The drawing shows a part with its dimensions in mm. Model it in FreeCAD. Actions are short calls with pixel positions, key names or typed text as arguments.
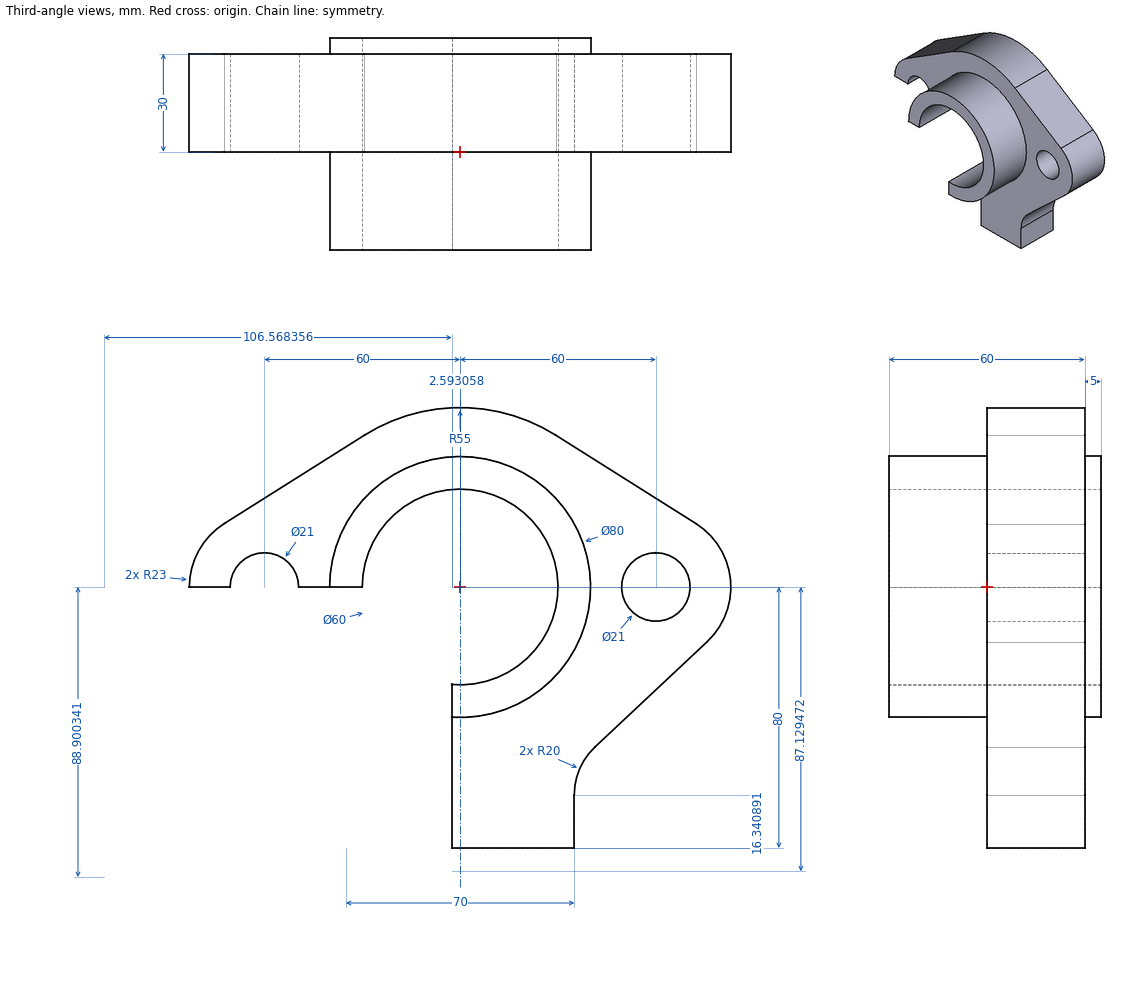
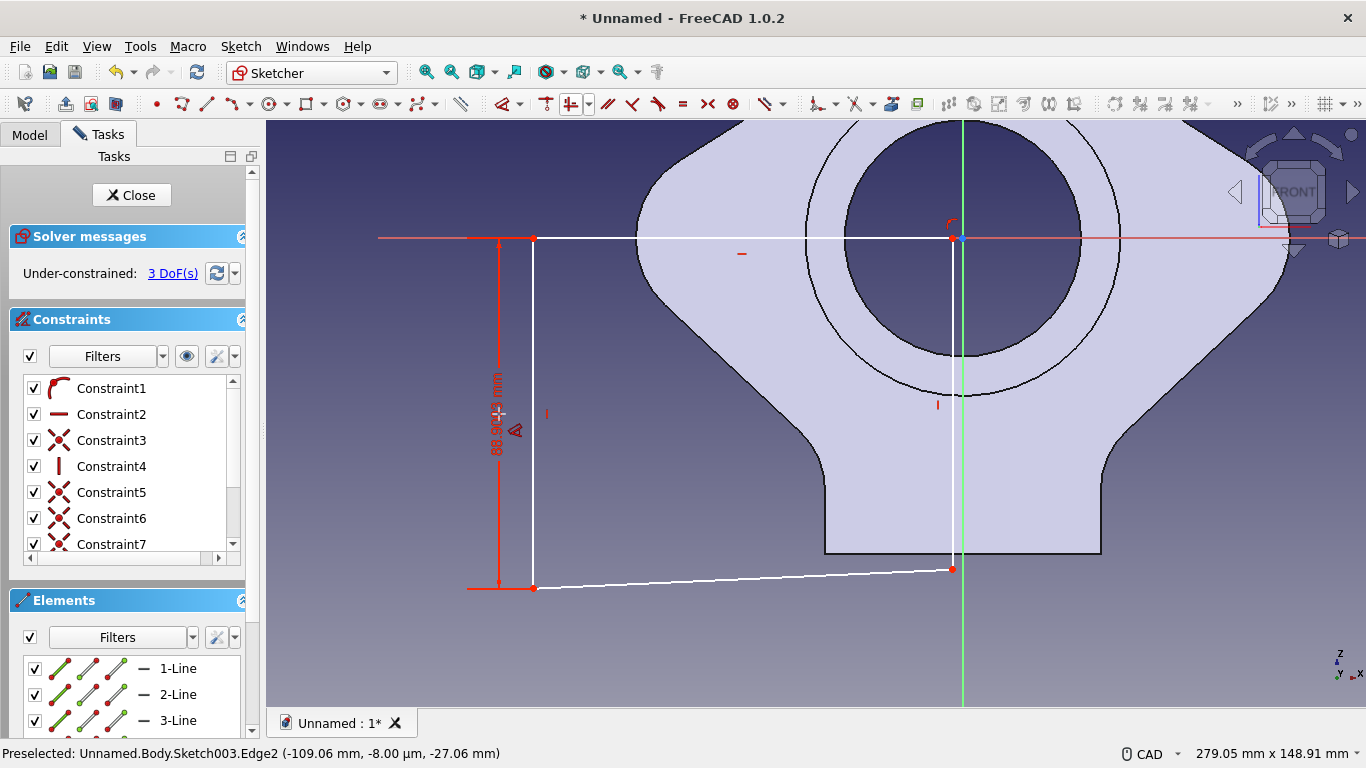
scroll(953, 470, up, 2)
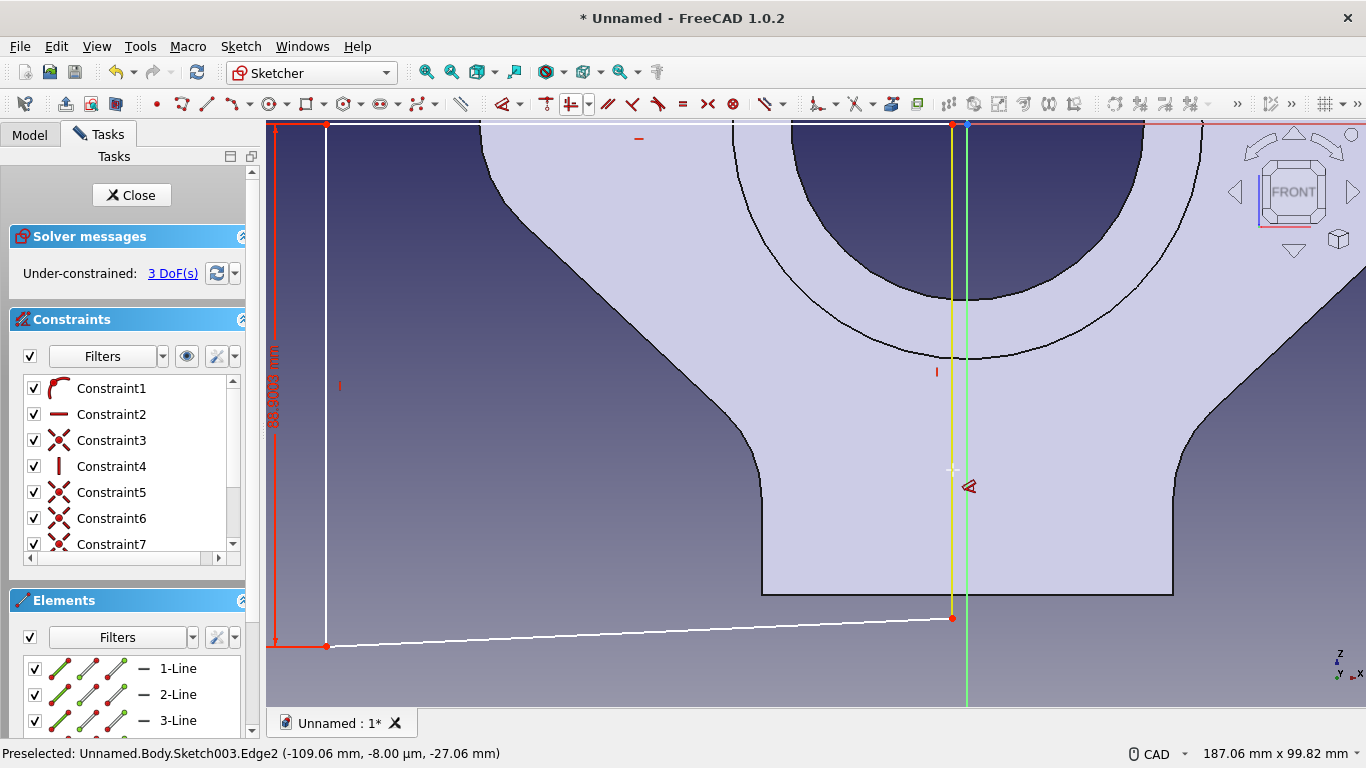
click(952, 470)
click(986, 383)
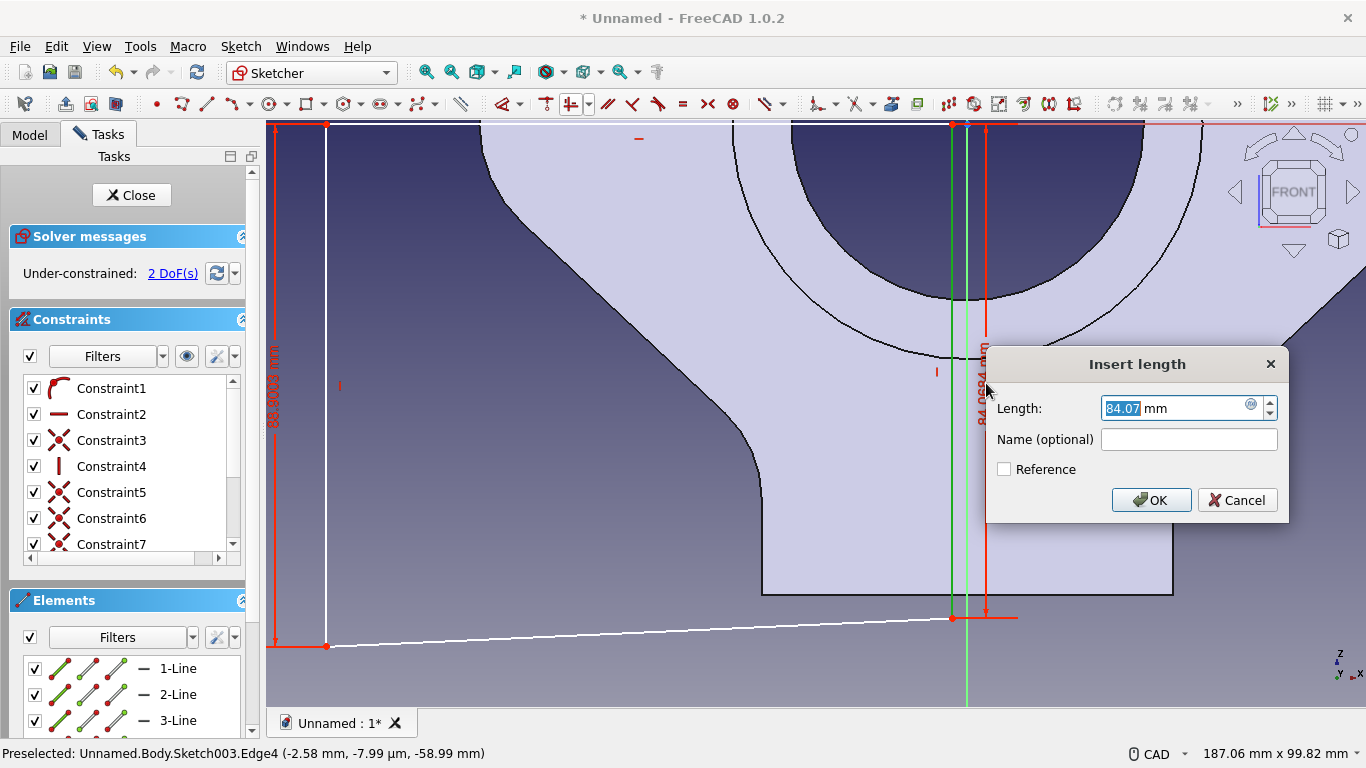
text(87.129472)
key(Return)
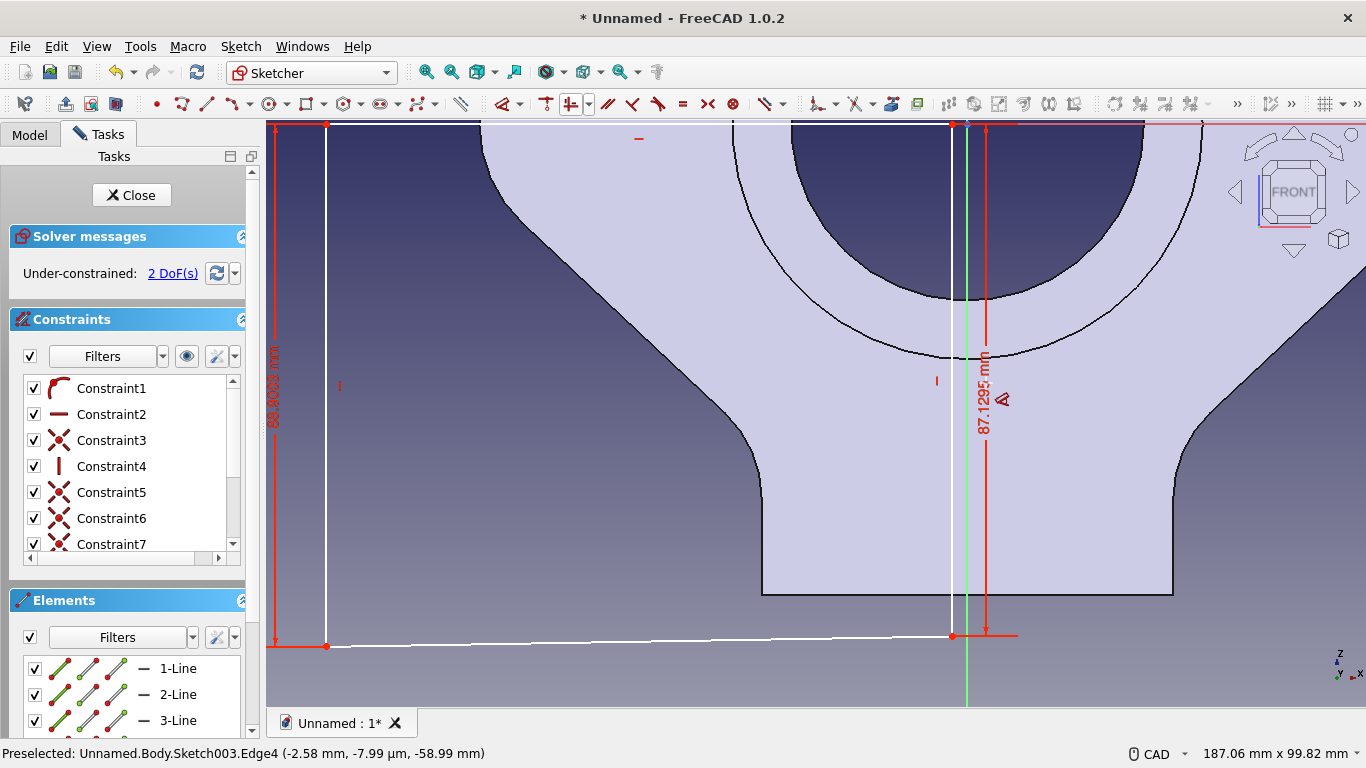
scroll(953, 470, down, 2)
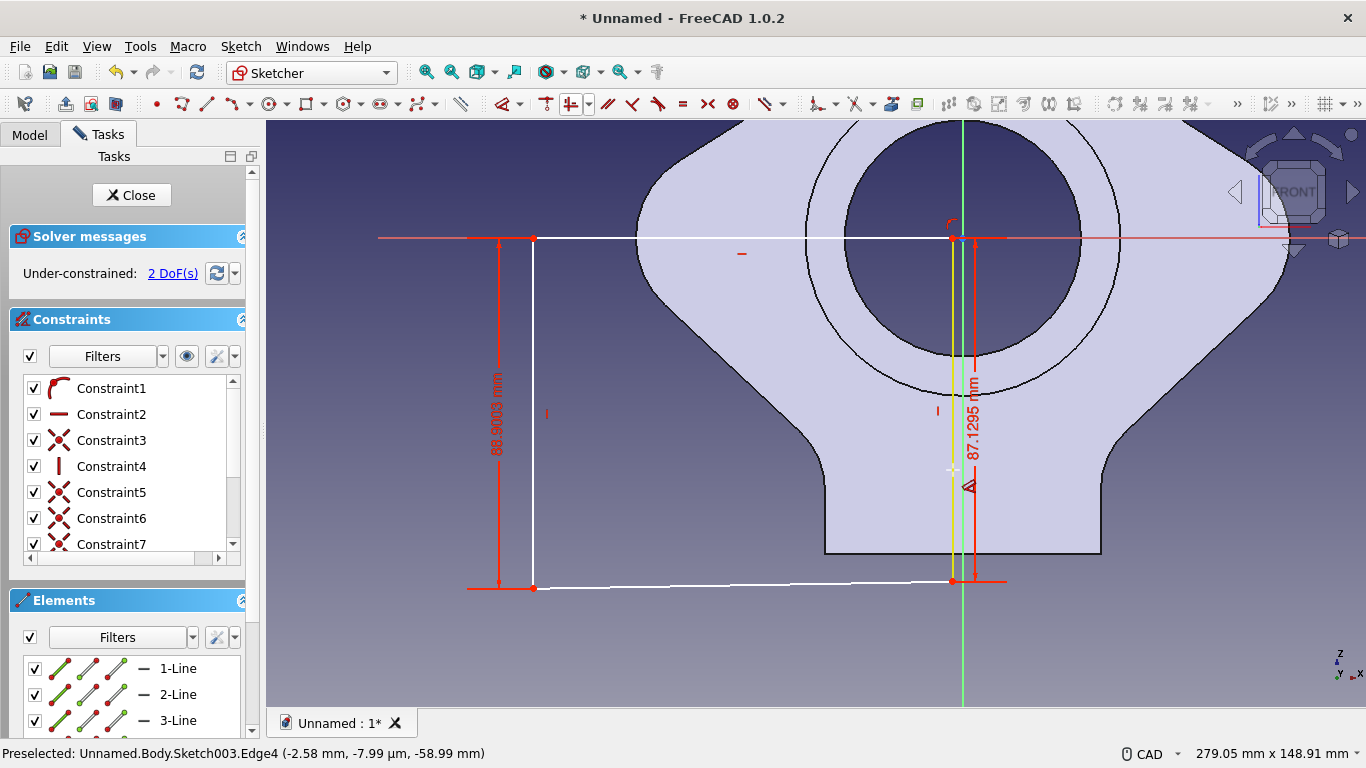
scroll(953, 238, up, 7)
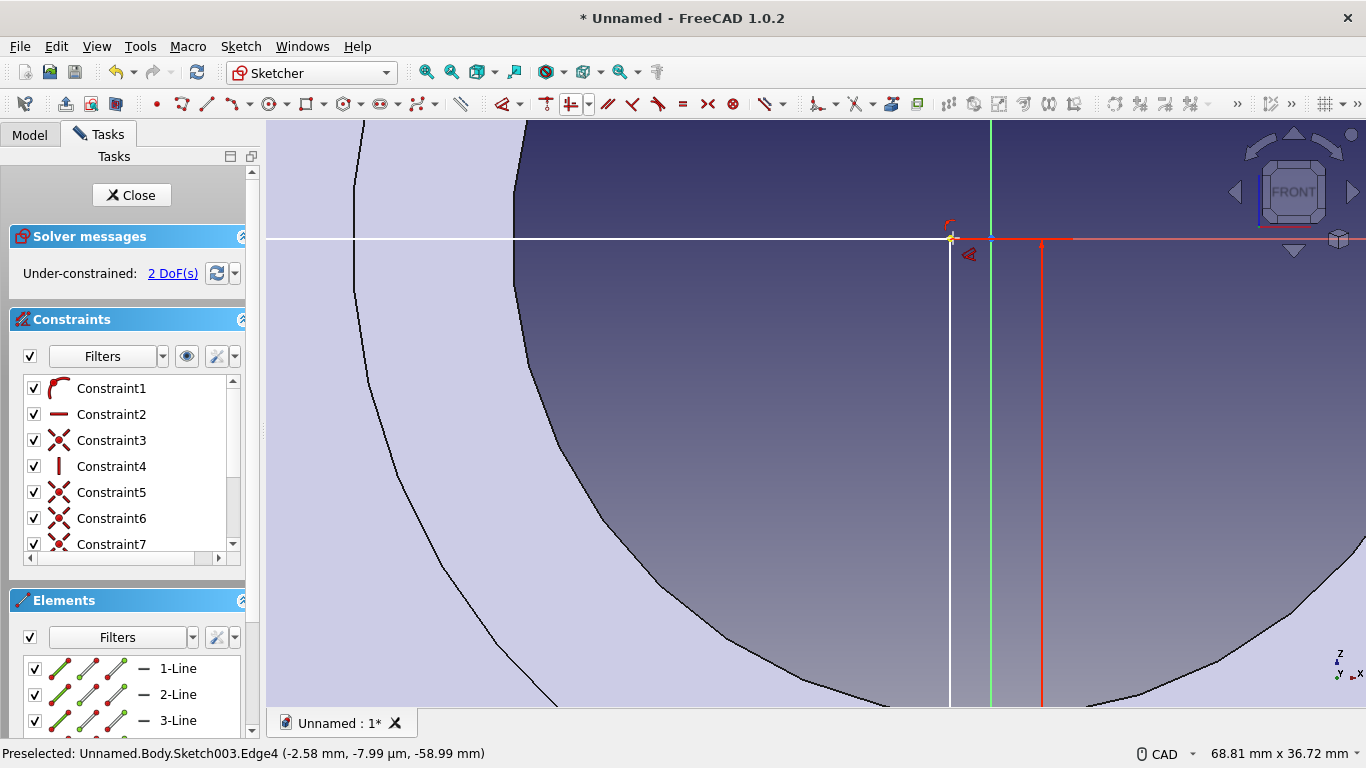
click(950, 239)
click(971, 205)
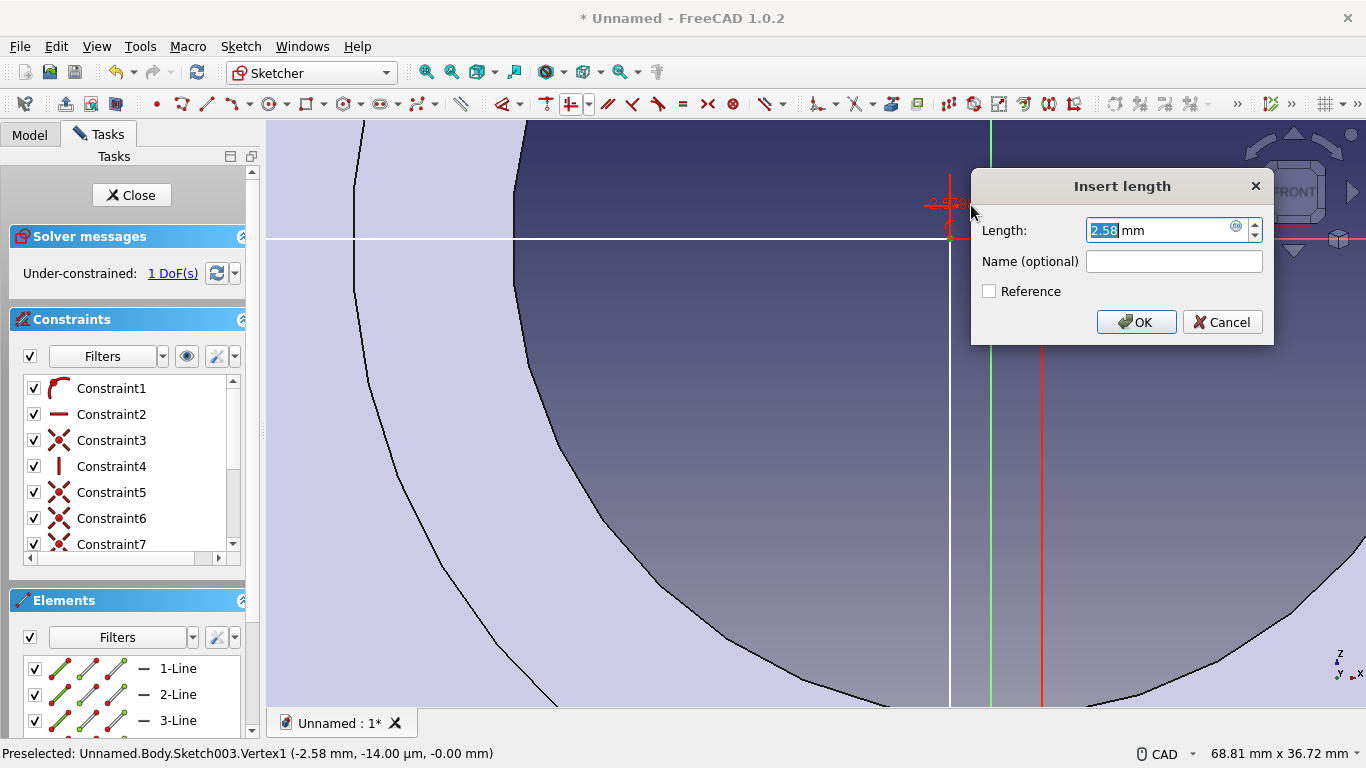
text(2.593058)
key(Return)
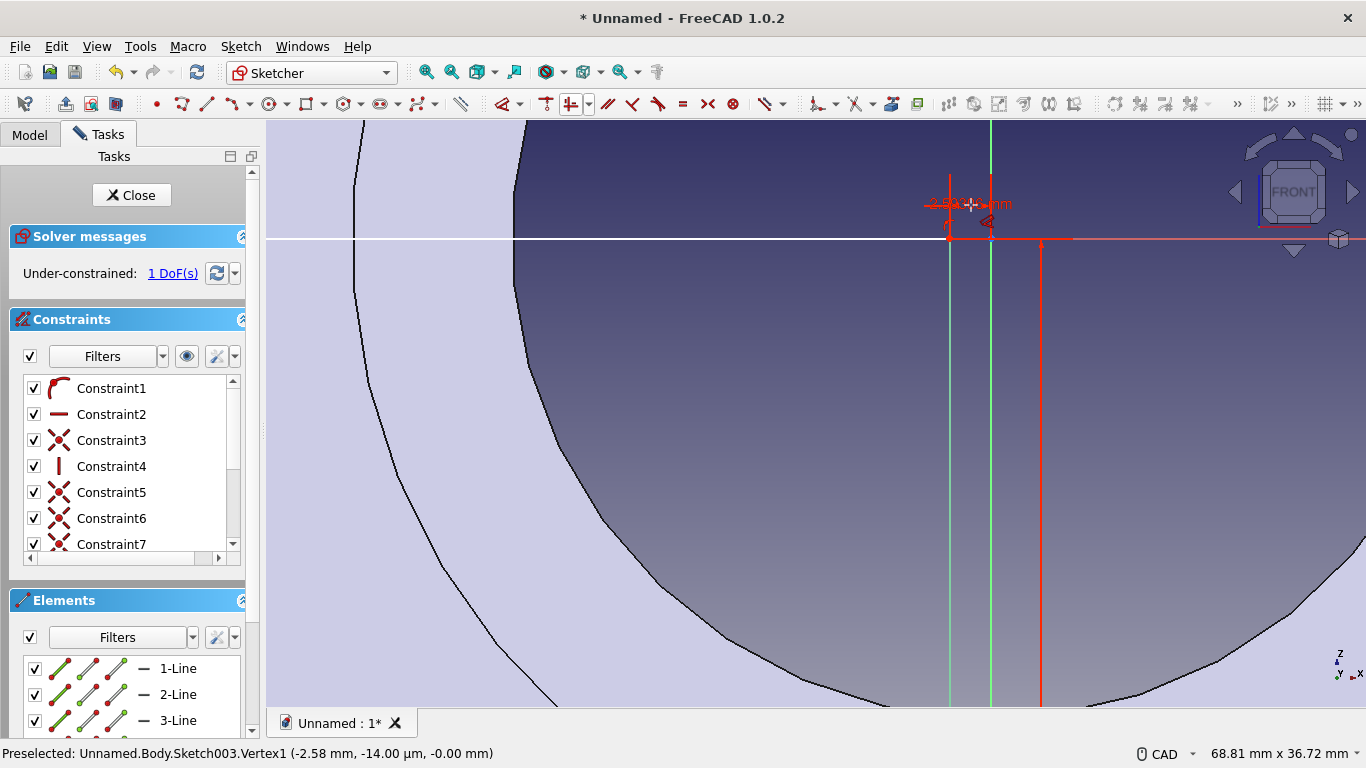
scroll(953, 238, down, 7)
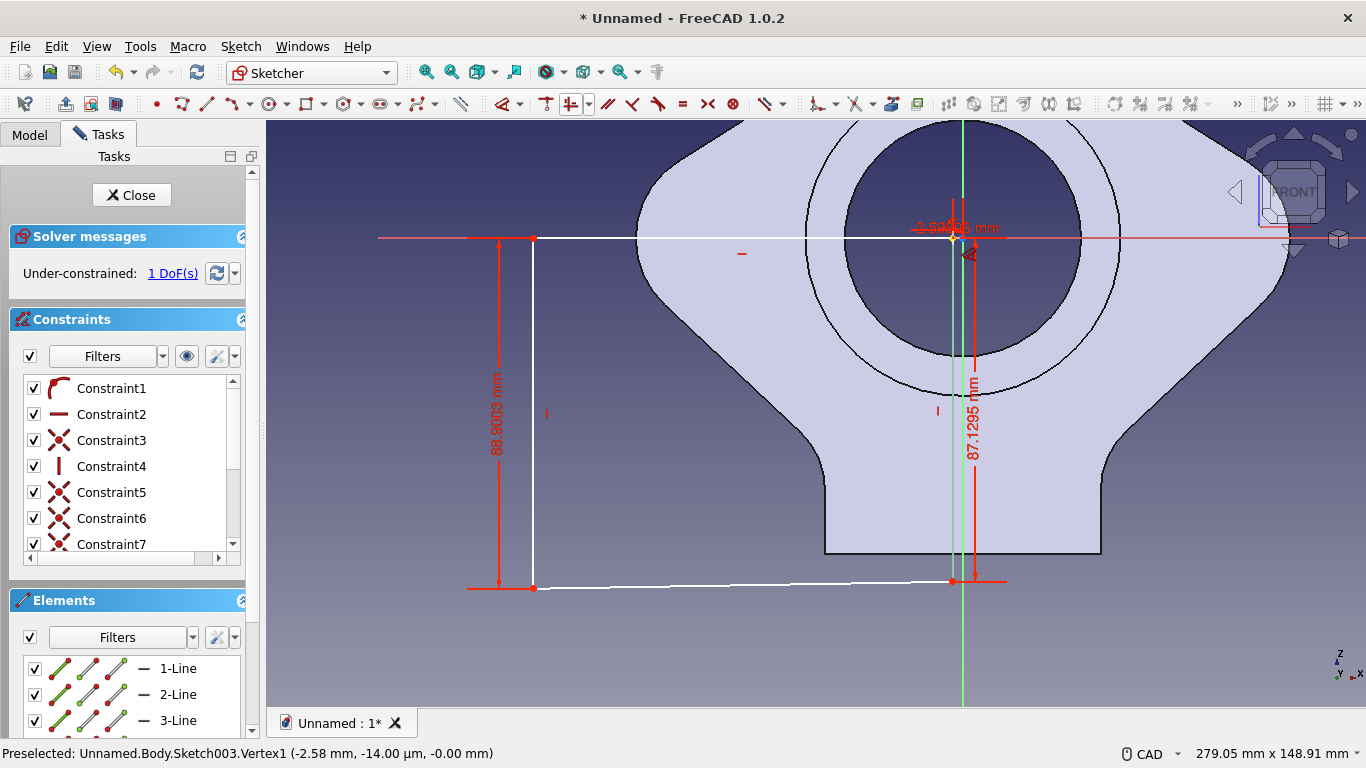
click(827, 238)
click(743, 204)